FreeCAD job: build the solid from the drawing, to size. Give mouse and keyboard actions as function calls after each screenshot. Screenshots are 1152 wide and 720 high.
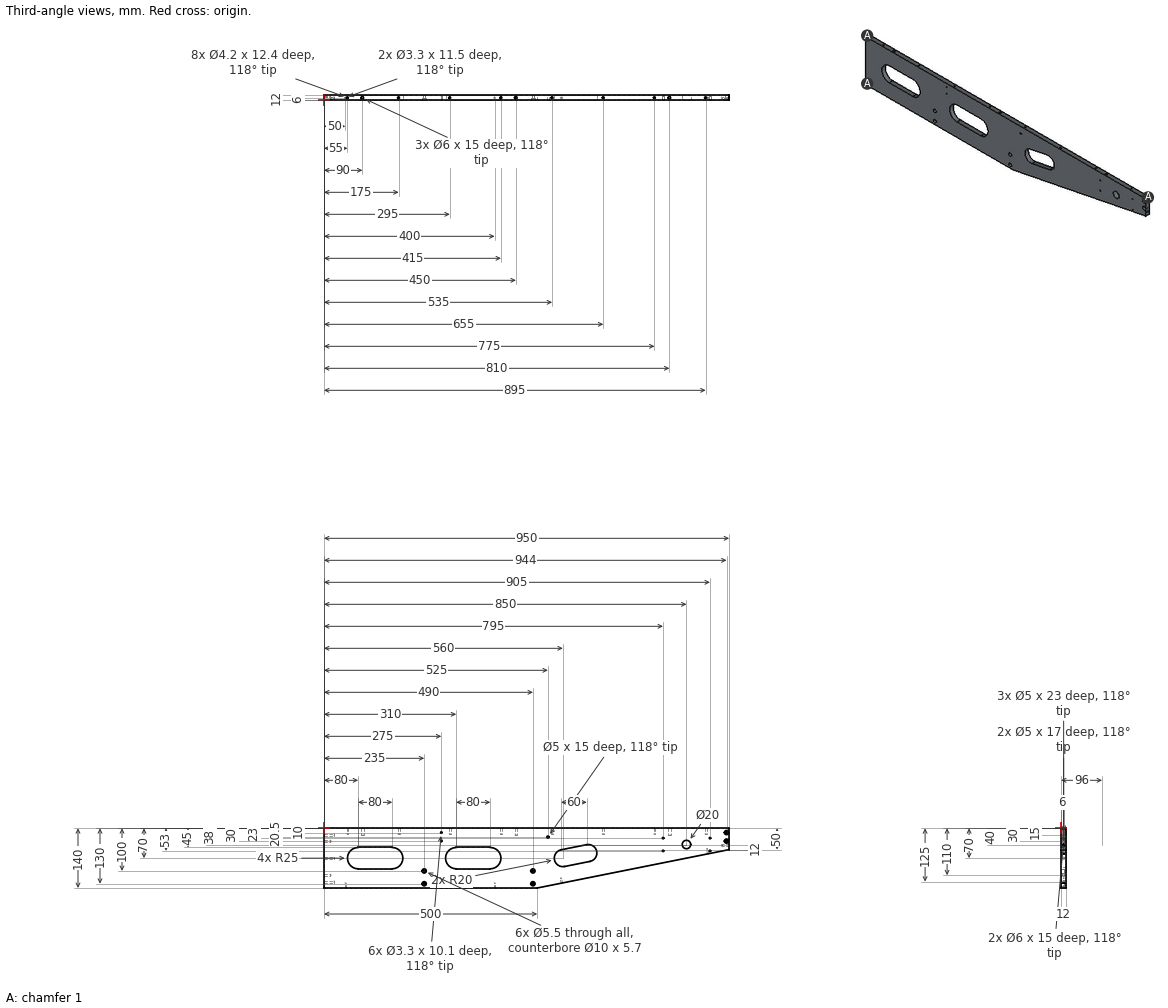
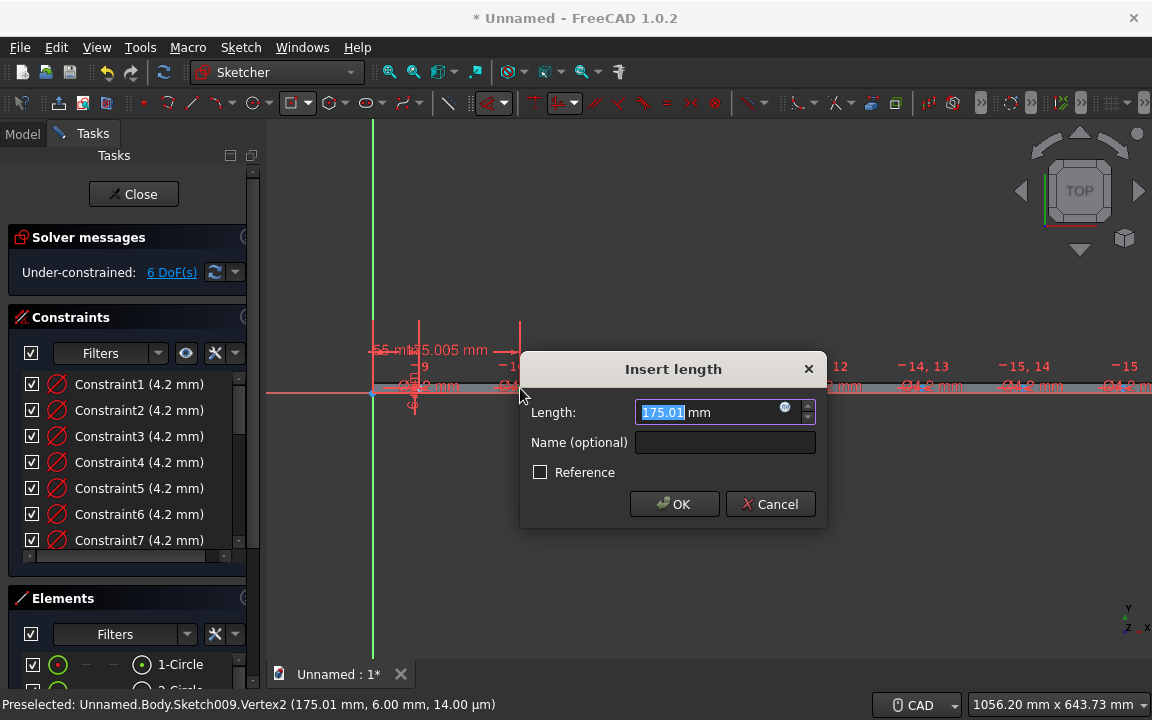
text(175)
key(Return)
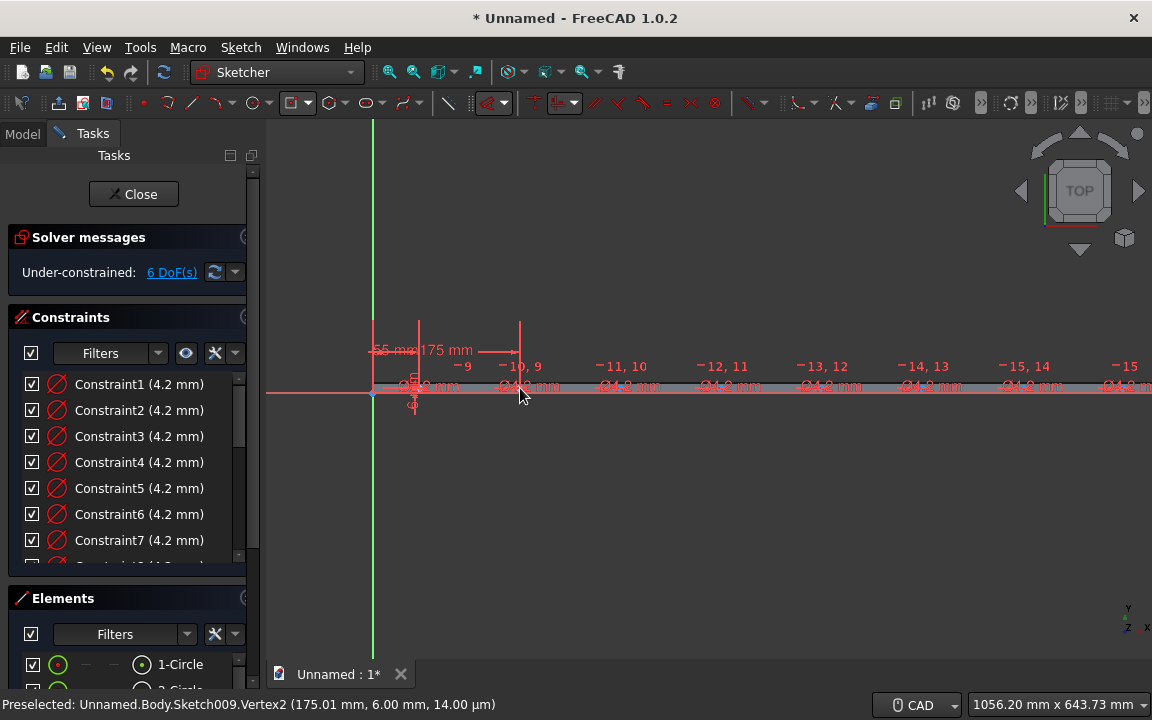
click(621, 388)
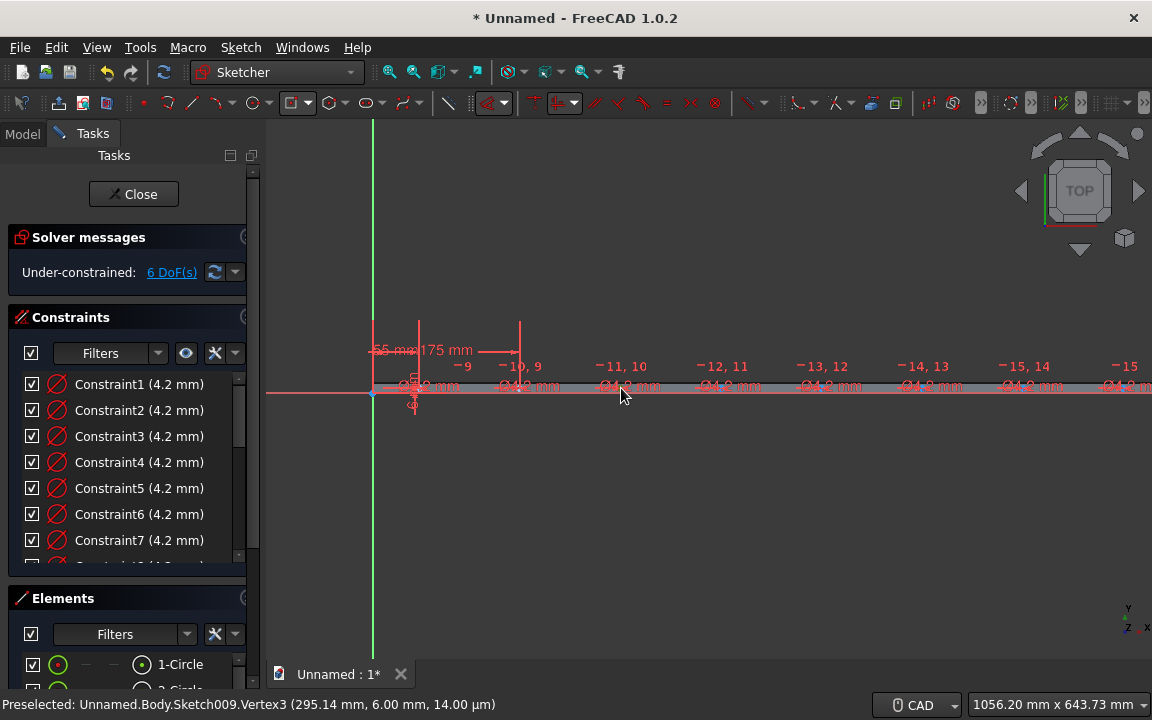
key(l)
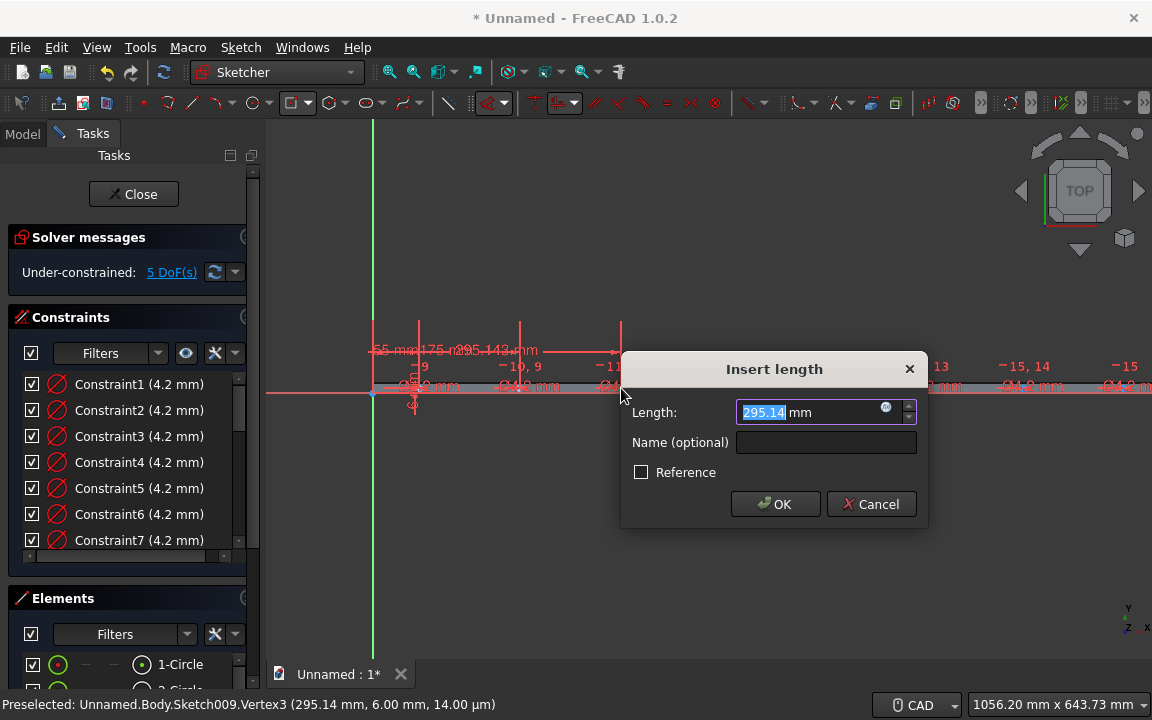
text(295)
key(Return)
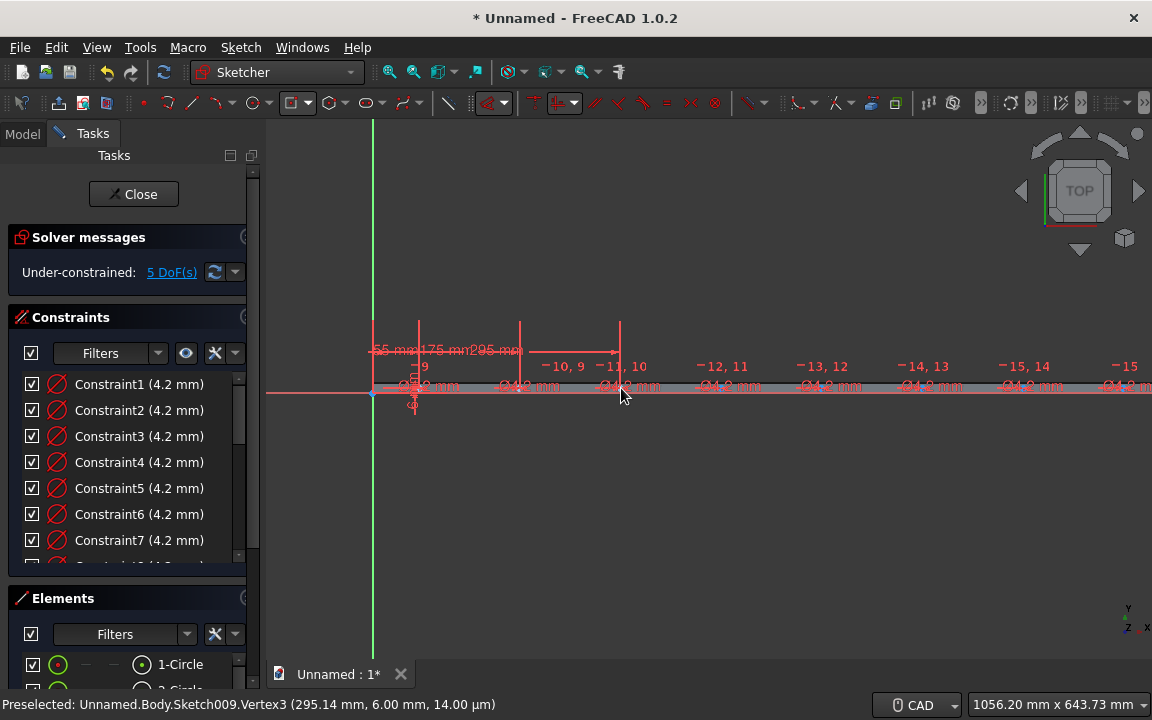
click(721, 388)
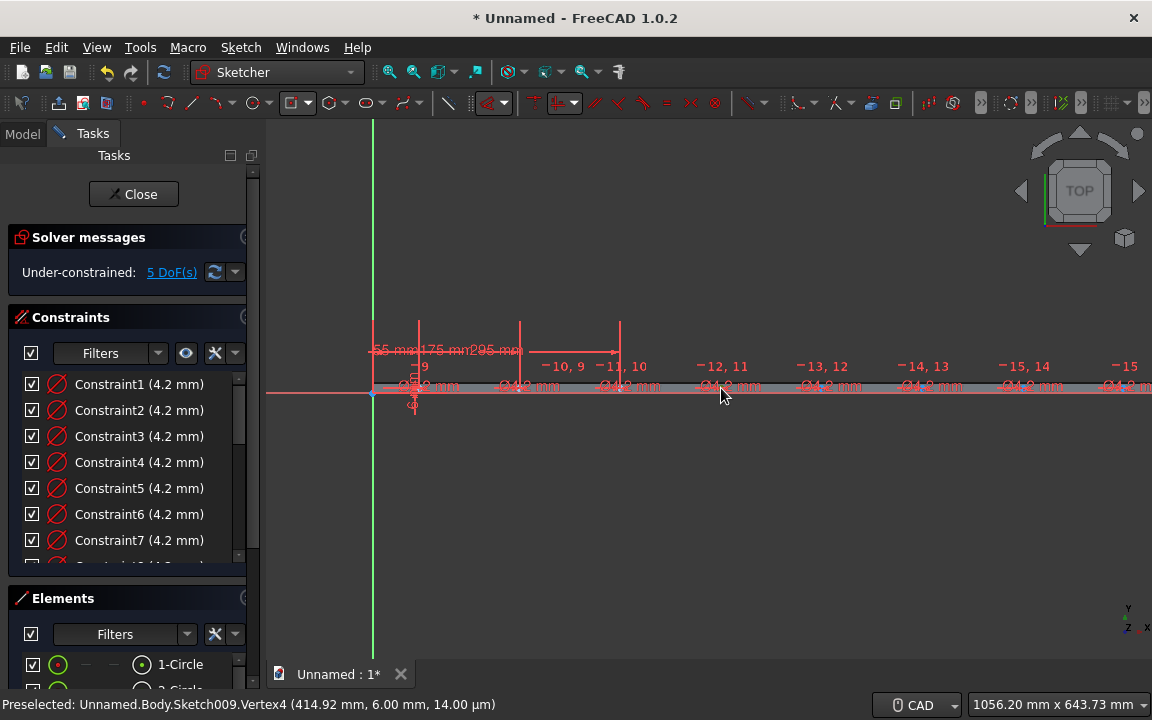
click(506, 104)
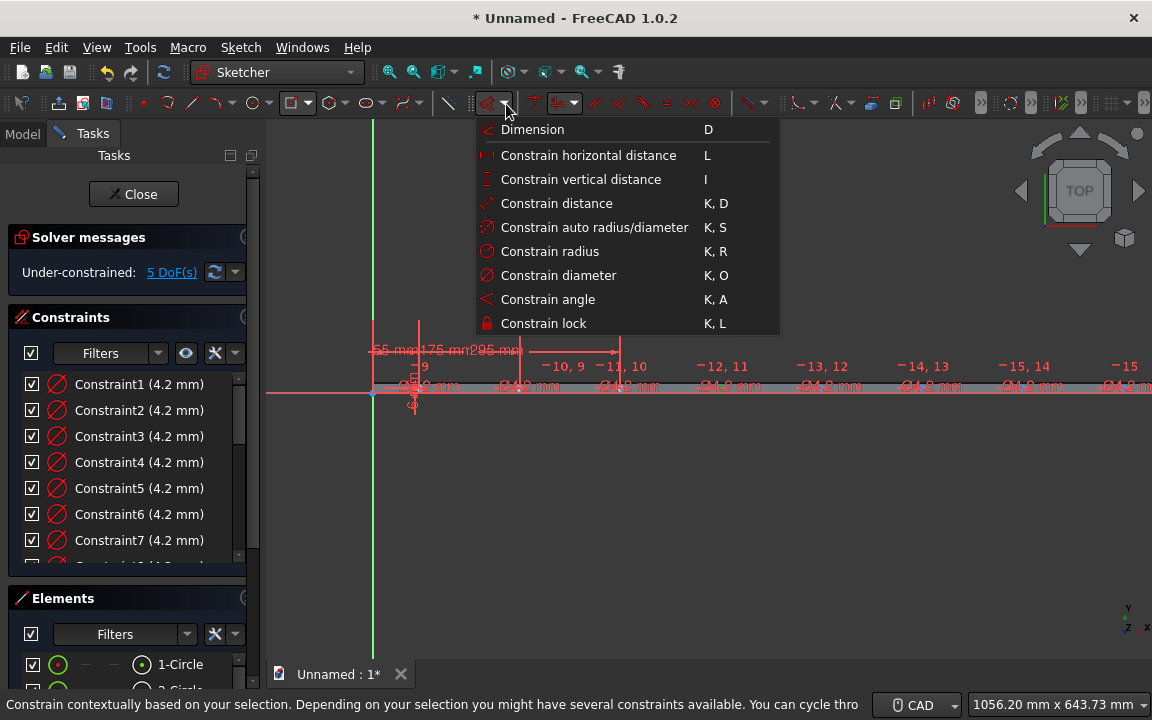
click(628, 155)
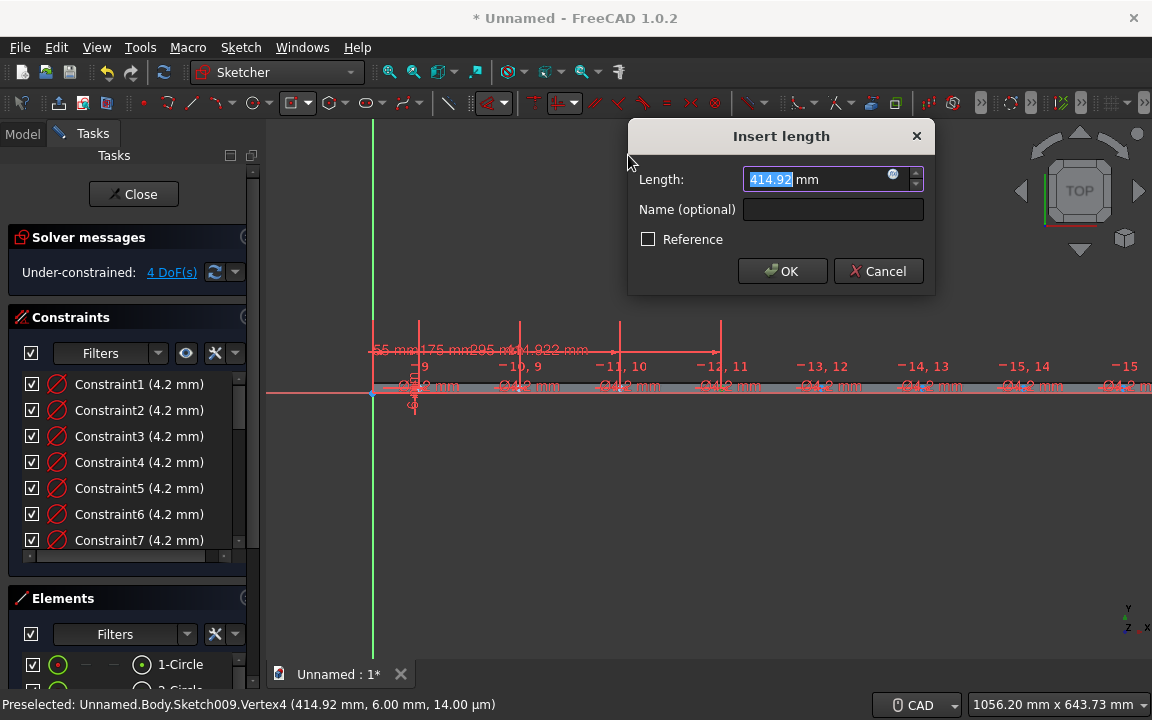
text(415)
key(Return)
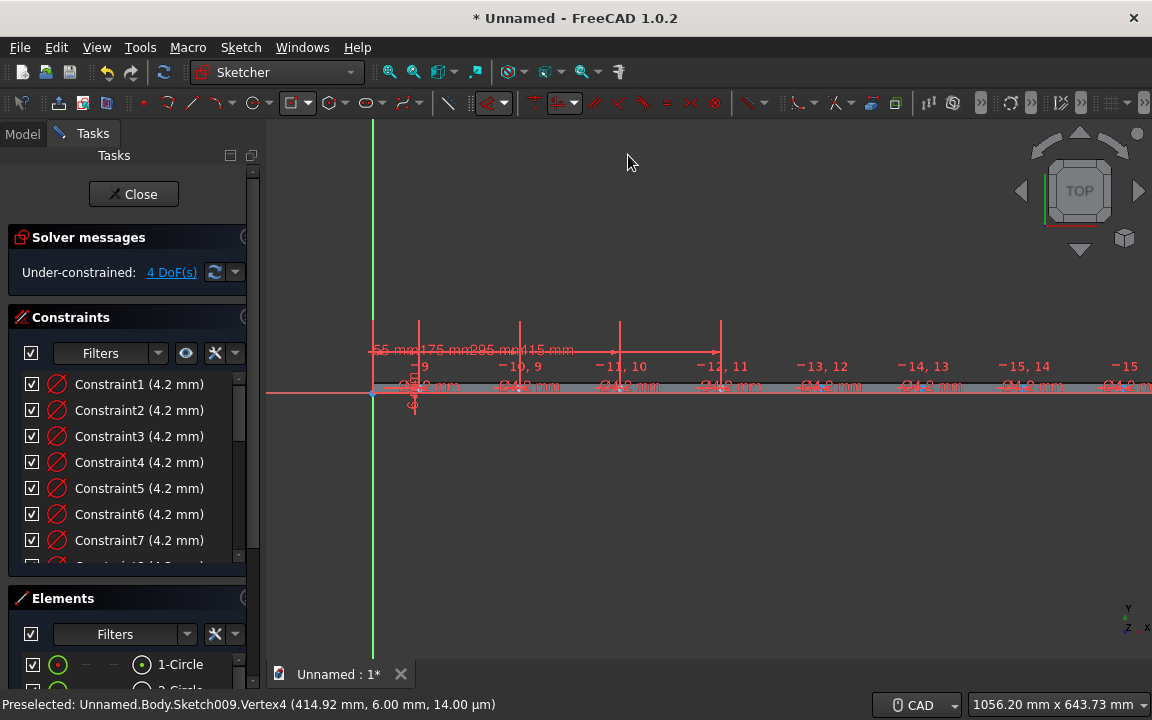
click(822, 388)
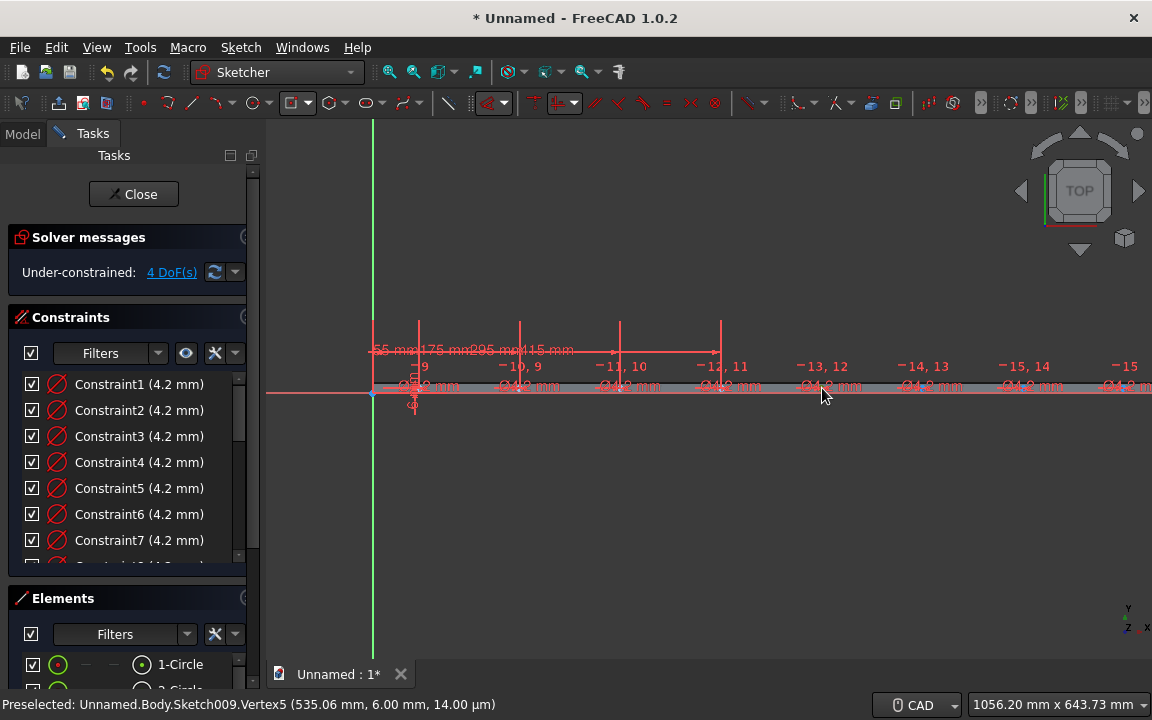
key(l)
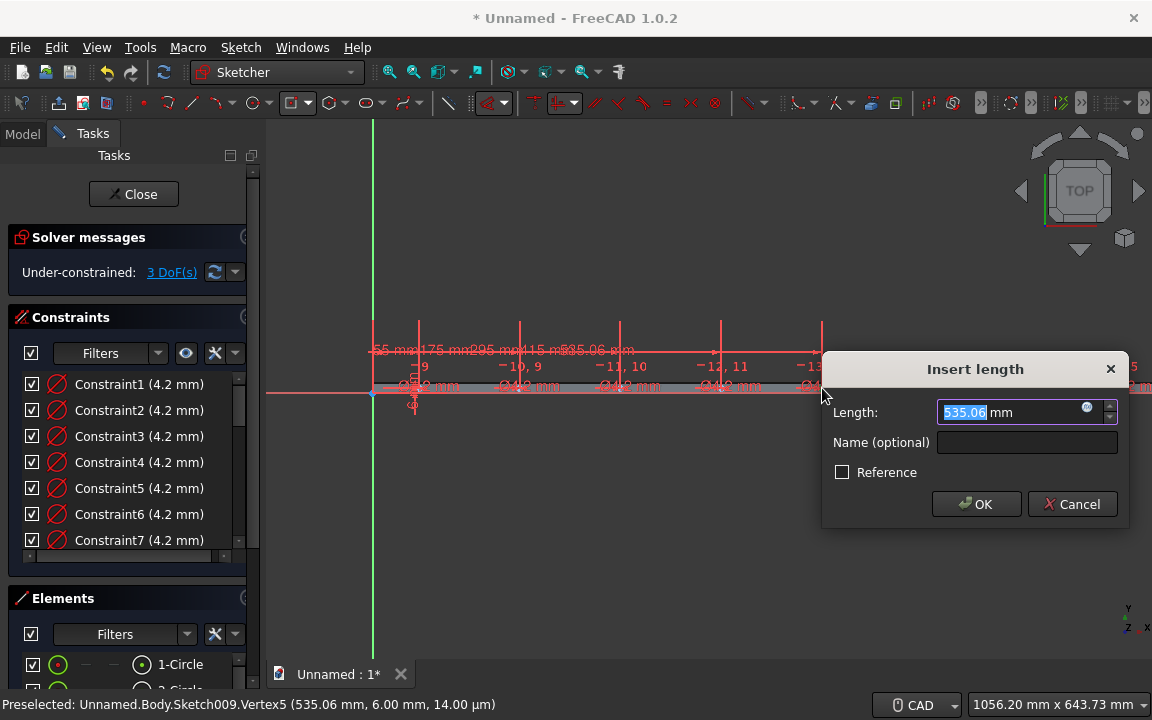
text(535)
key(Return)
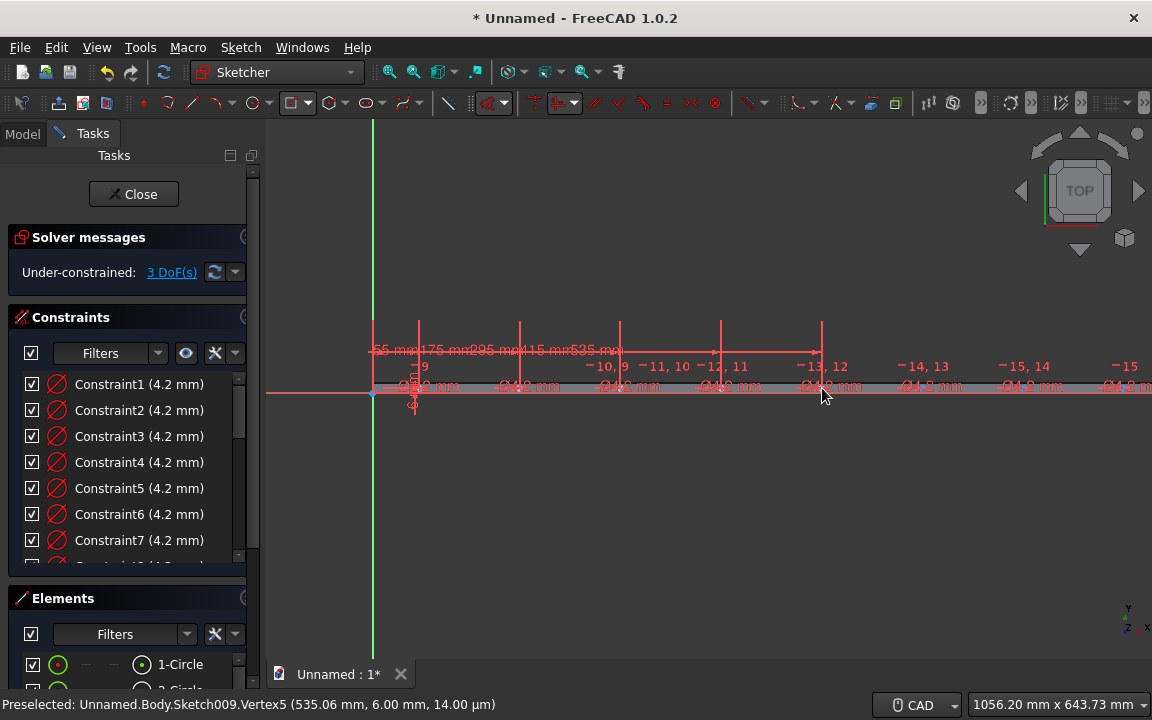
click(922, 388)